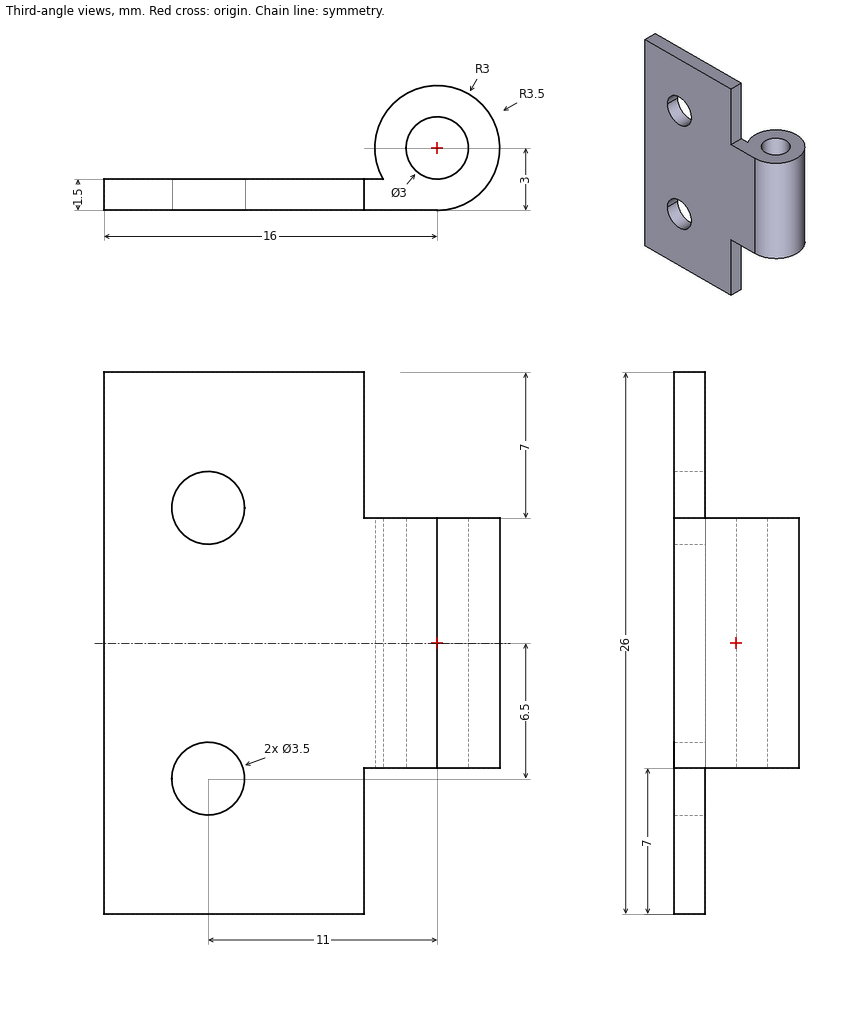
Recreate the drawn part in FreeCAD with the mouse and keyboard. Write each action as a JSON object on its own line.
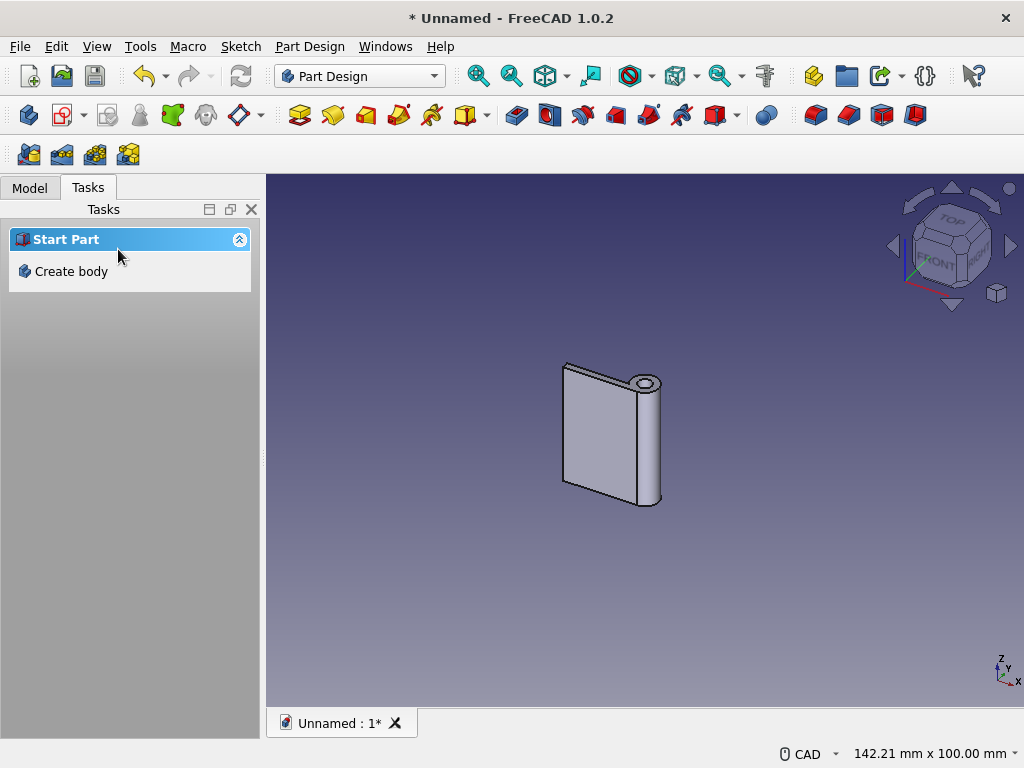
{"action": "left_click", "coordinate": [479, 76]}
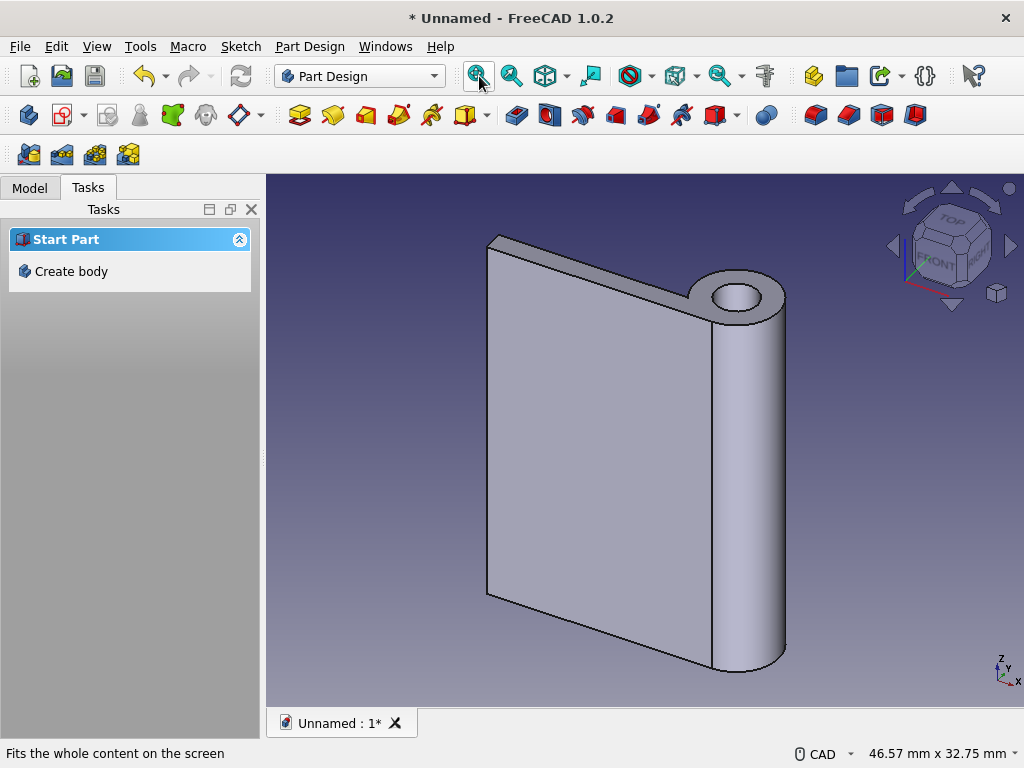
{"action": "left_click", "coordinate": [774, 290]}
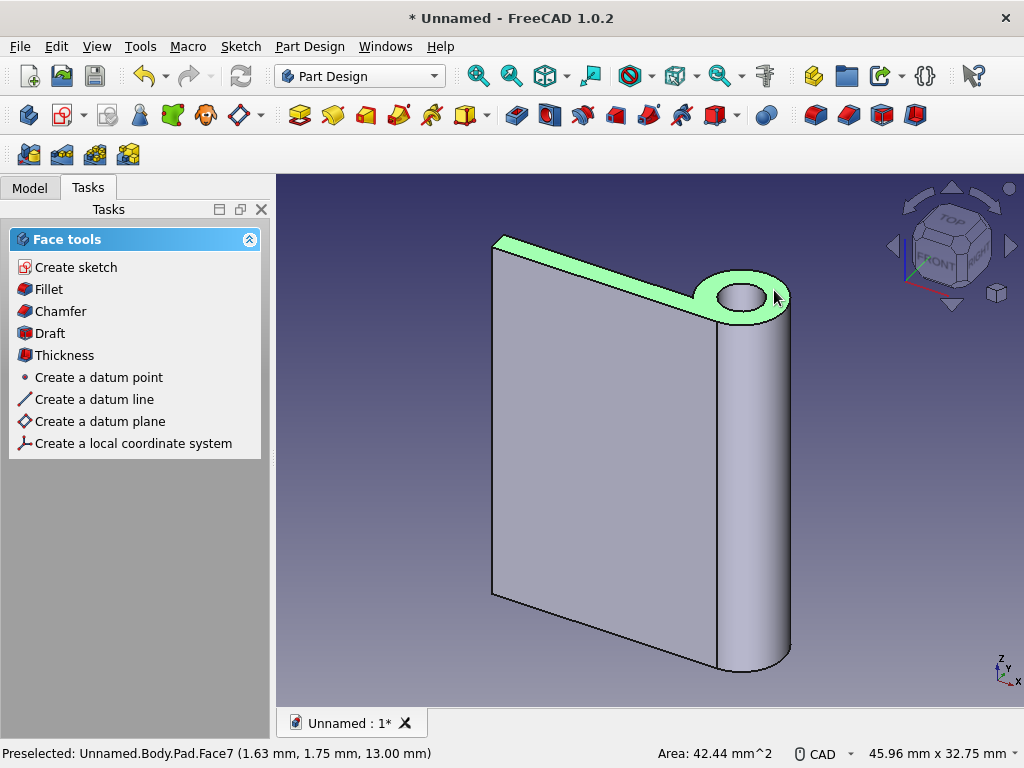
{"action": "left_click", "coordinate": [62, 116]}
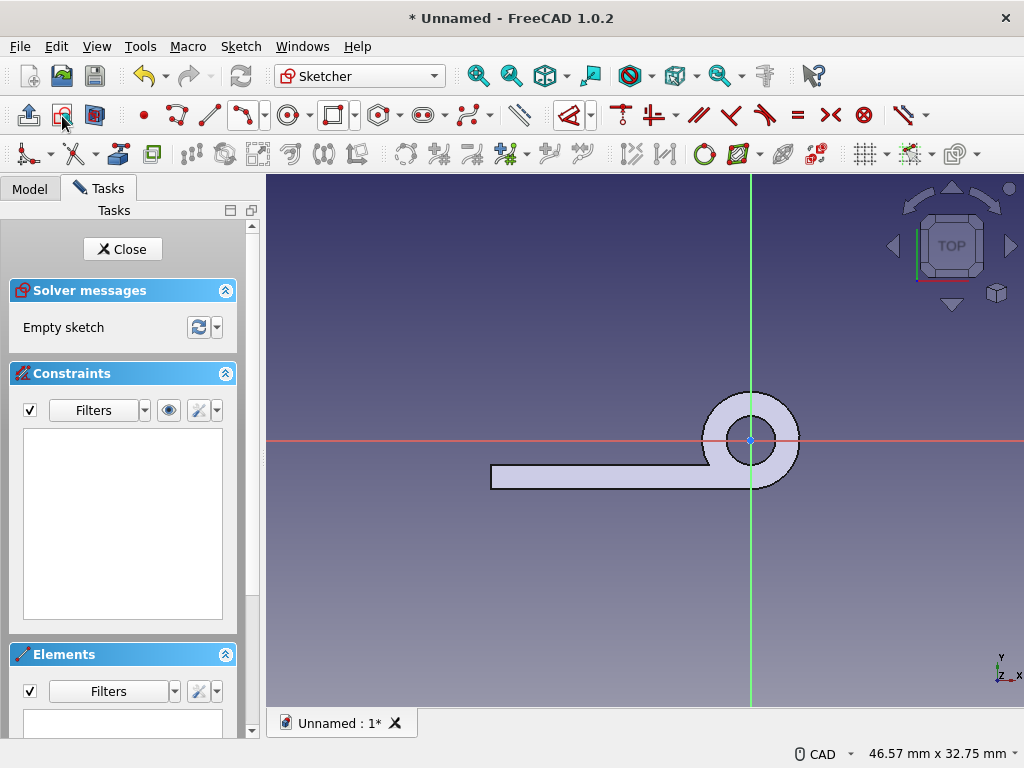
{"action": "scroll", "coordinate": [803, 454], "scroll_direction": "up", "scroll_amount": 7}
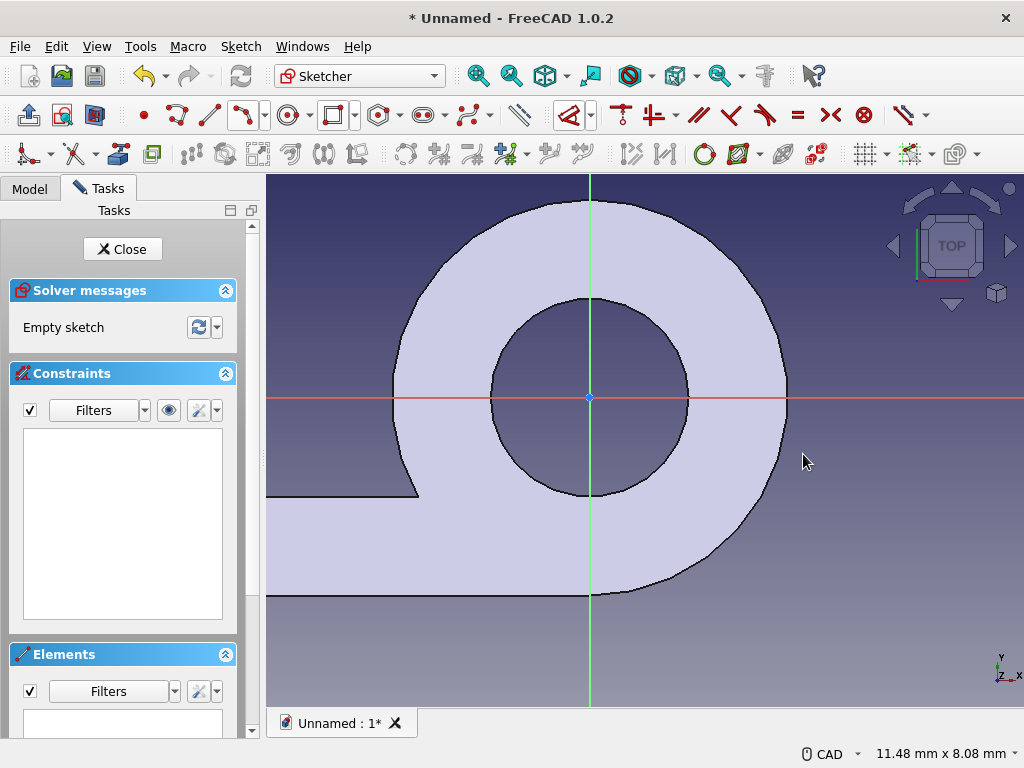
{"action": "left_click", "coordinate": [177, 116]}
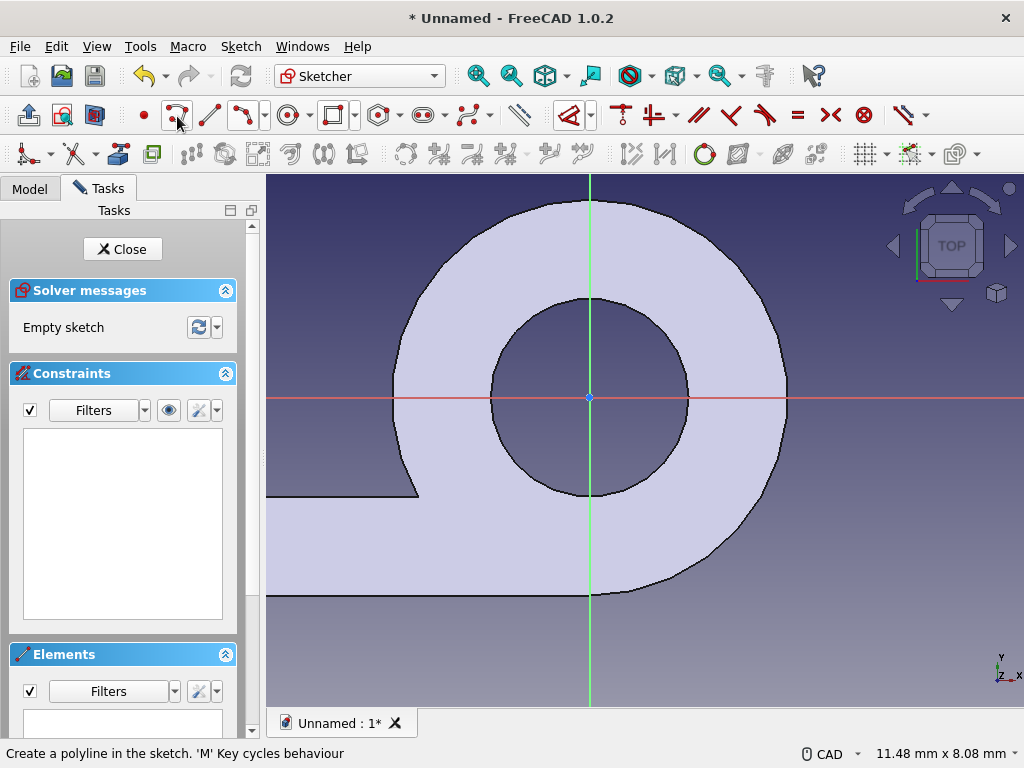
{"action": "left_click", "coordinate": [359, 398]}
{"action": "left_click", "coordinate": [359, 596]}
{"action": "left_click", "coordinate": [471, 596]}
{"action": "right_click", "coordinate": [471, 596]}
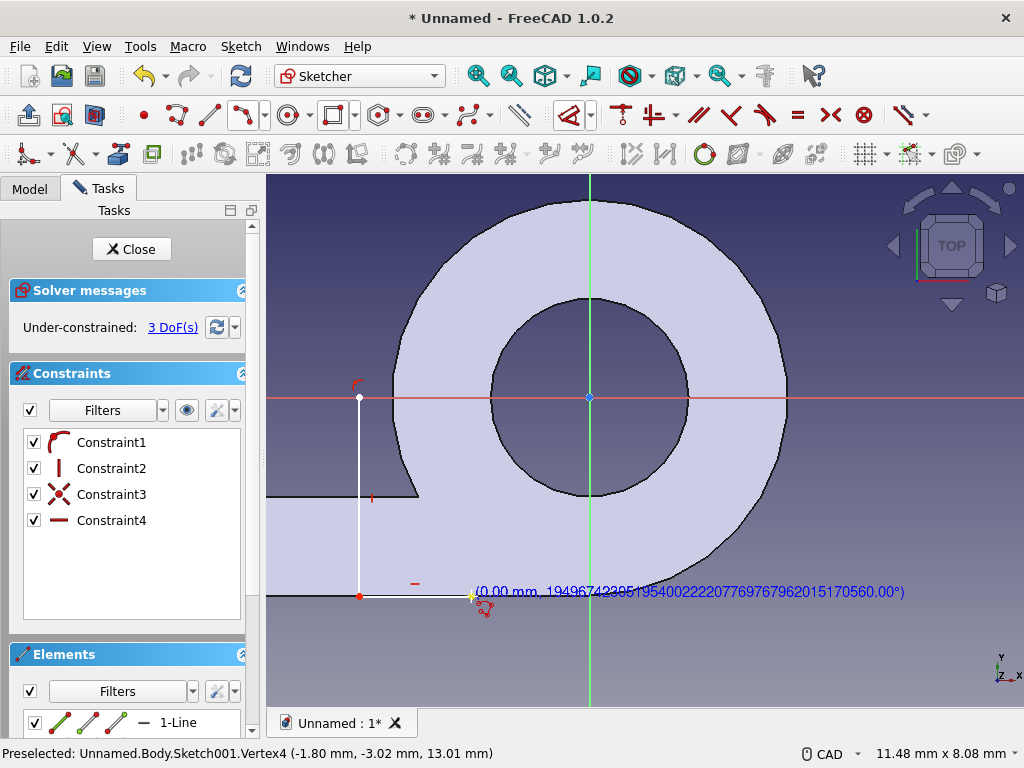
{"action": "left_click", "coordinate": [242, 116]}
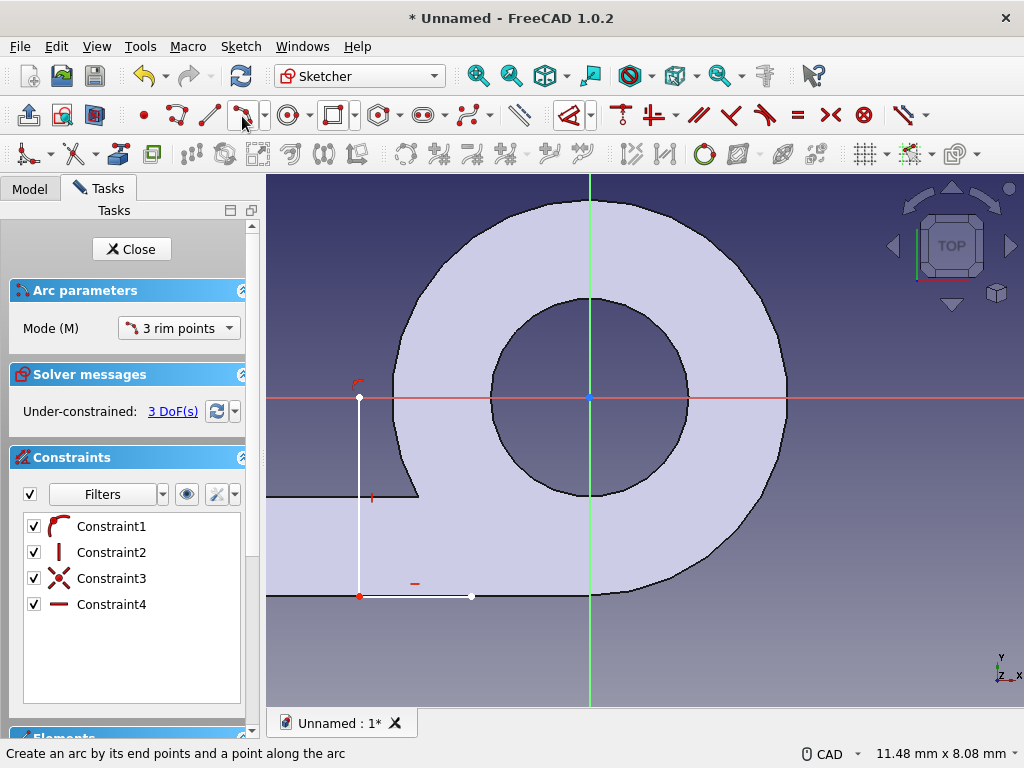
{"action": "left_click", "coordinate": [471, 597]}
{"action": "left_click", "coordinate": [359, 398]}
{"action": "left_click", "coordinate": [791, 284]}
{"action": "key", "text": "Escape"}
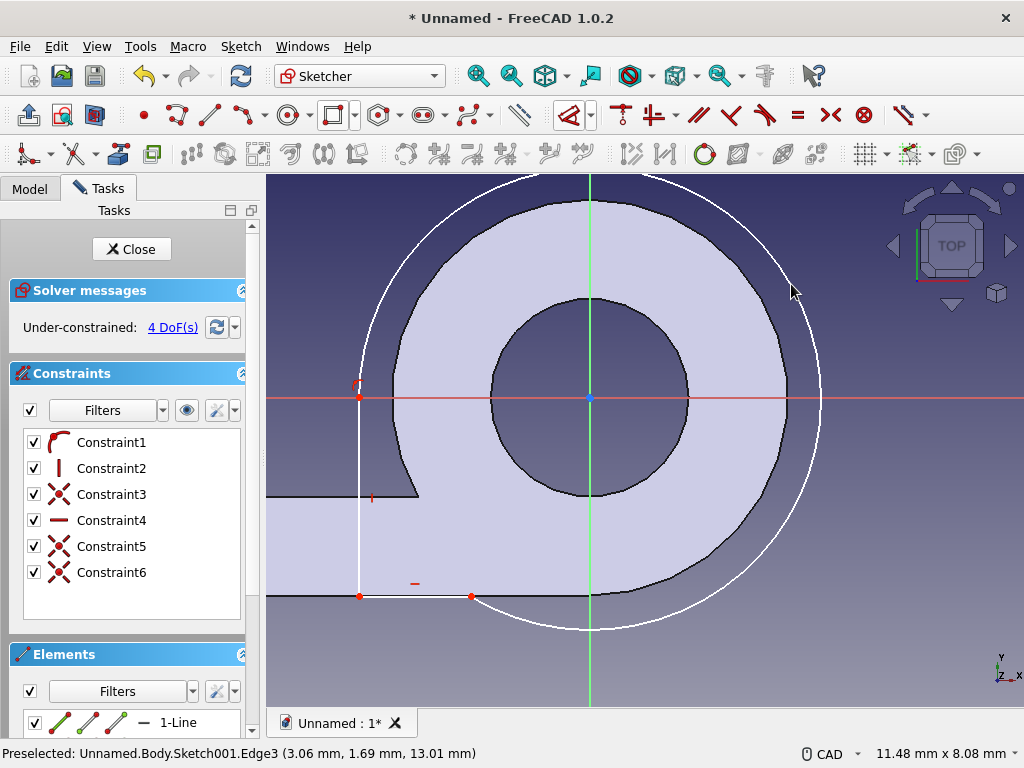
{"action": "left_click", "coordinate": [359, 457]}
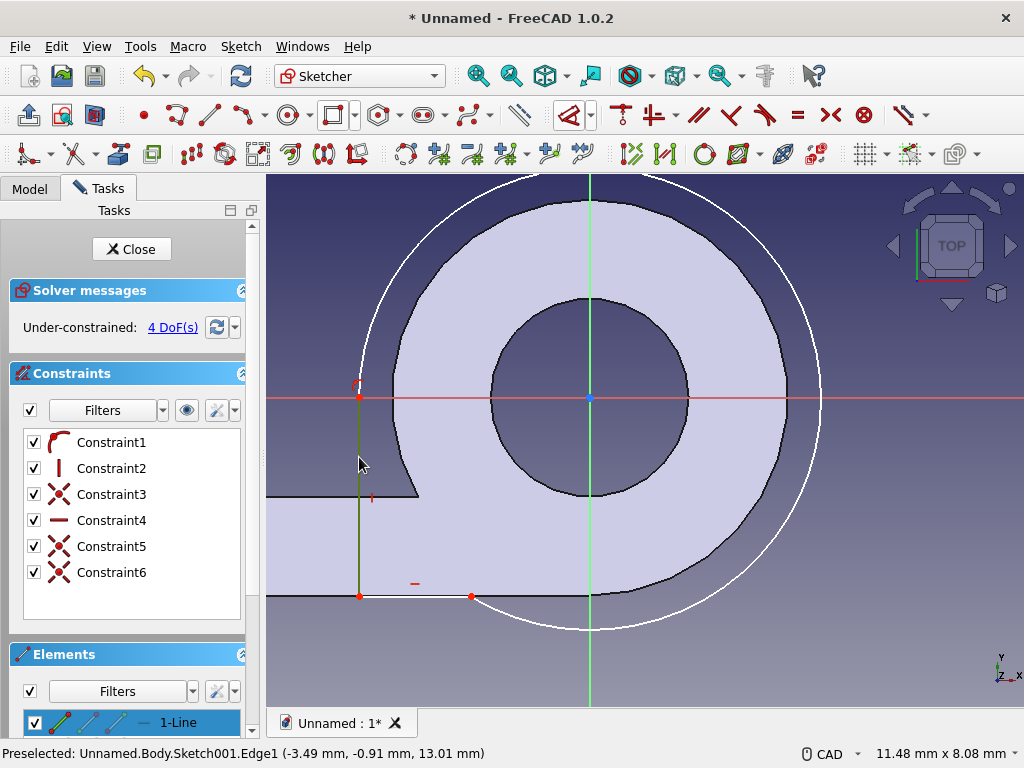
{"action": "left_click", "coordinate": [788, 517]}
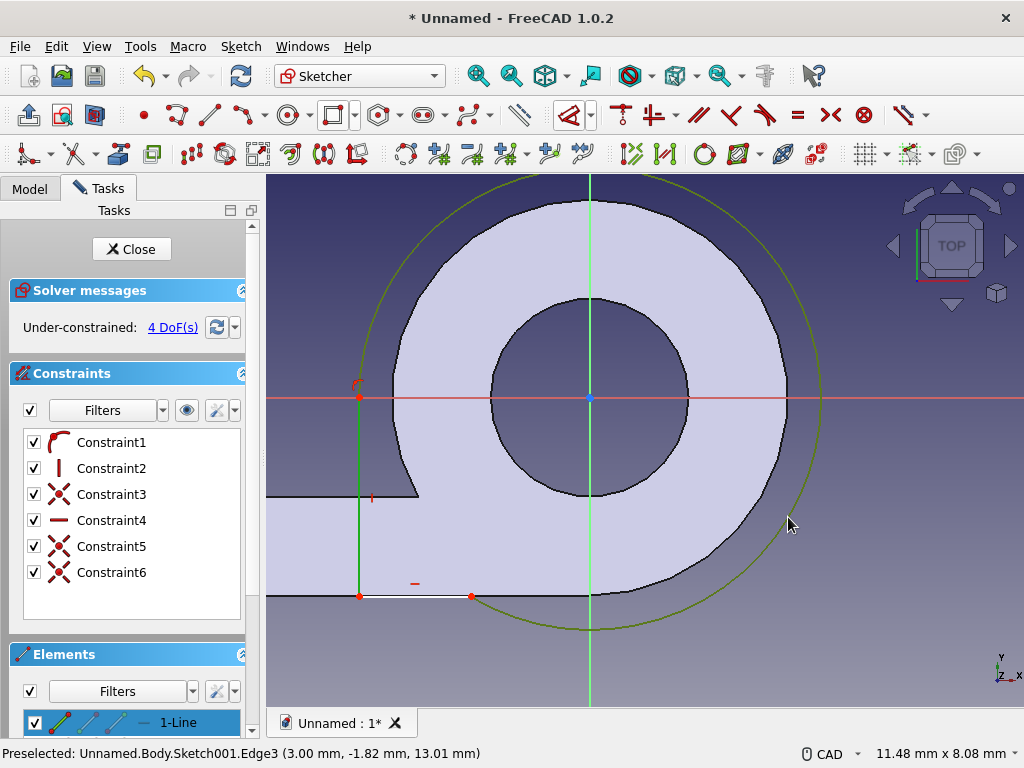
{"action": "key", "text": "t"}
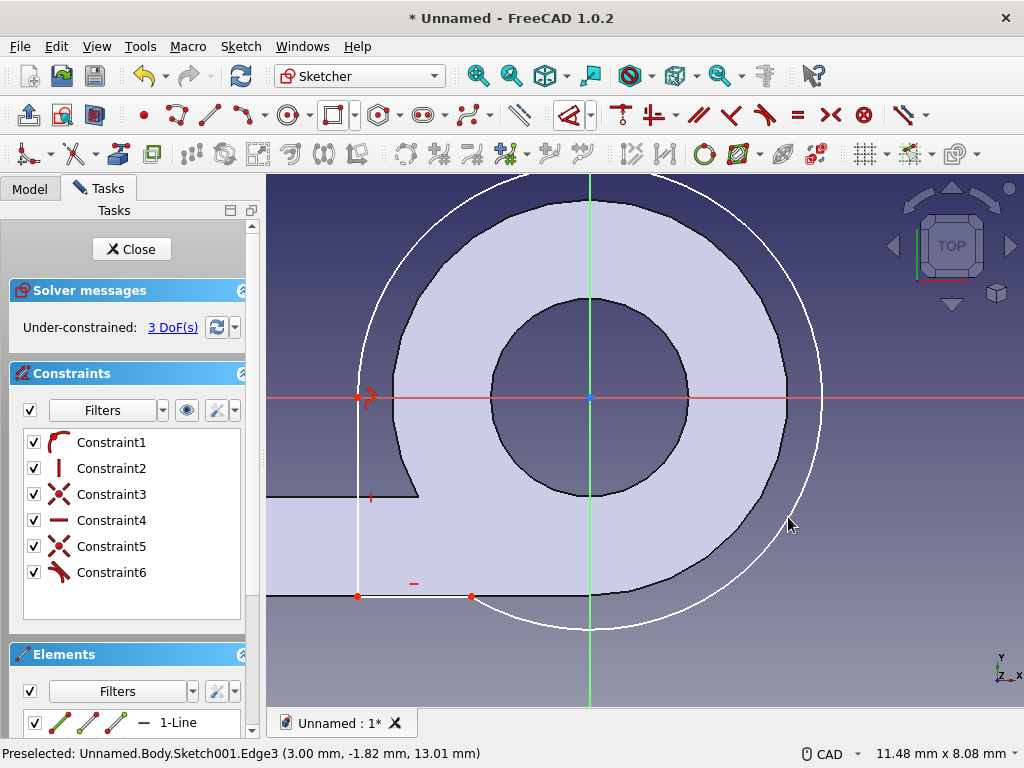
{"action": "left_click", "coordinate": [590, 398]}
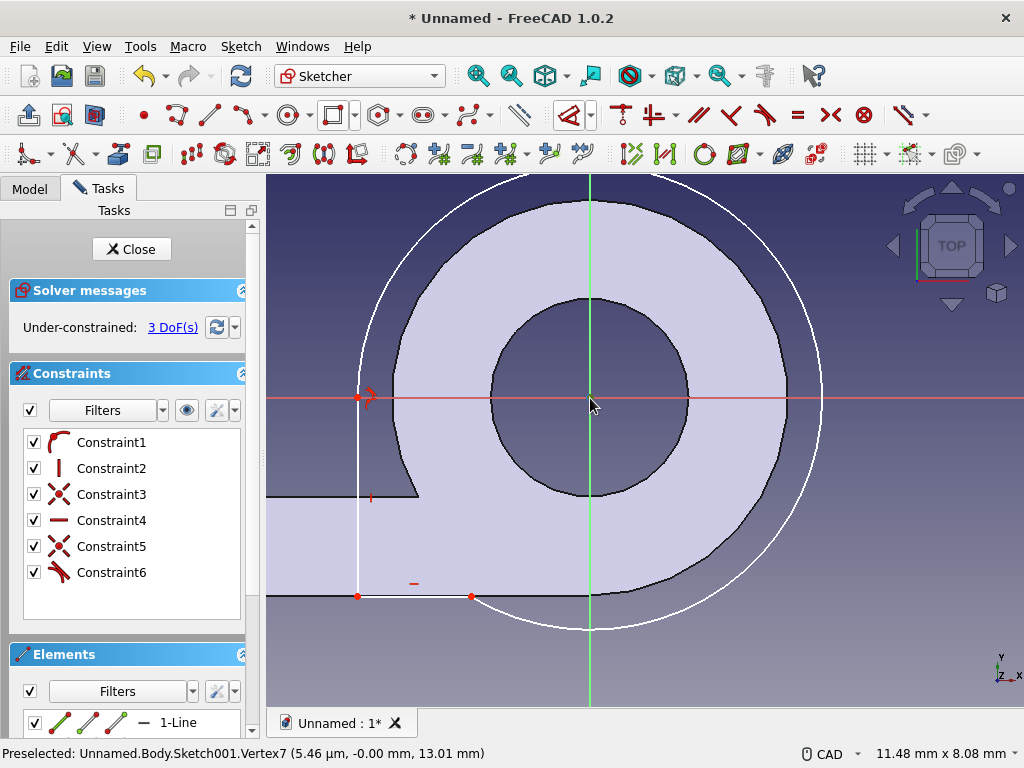
{"action": "left_click", "coordinate": [590, 577]}